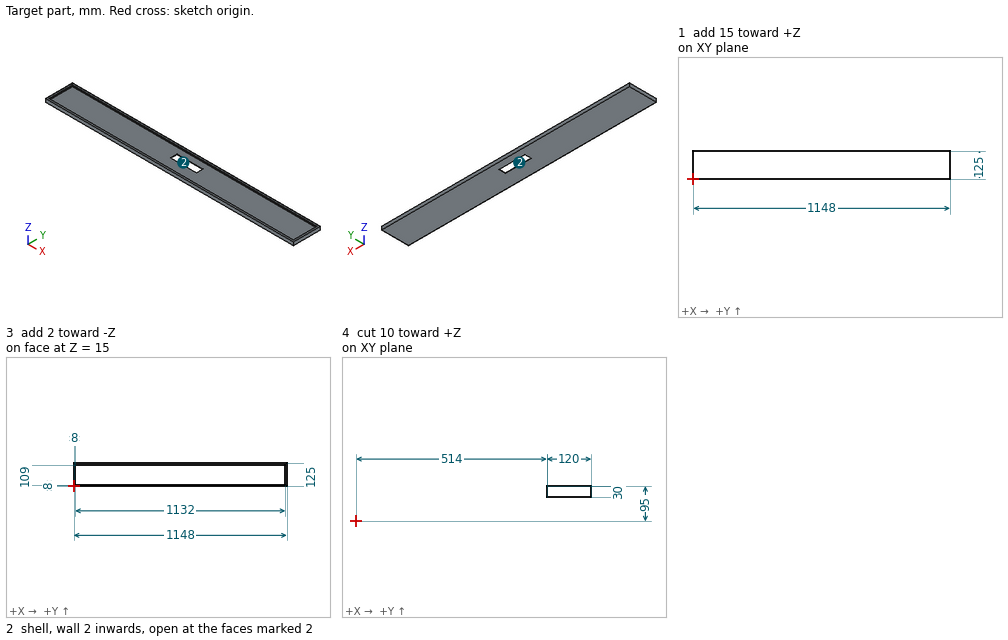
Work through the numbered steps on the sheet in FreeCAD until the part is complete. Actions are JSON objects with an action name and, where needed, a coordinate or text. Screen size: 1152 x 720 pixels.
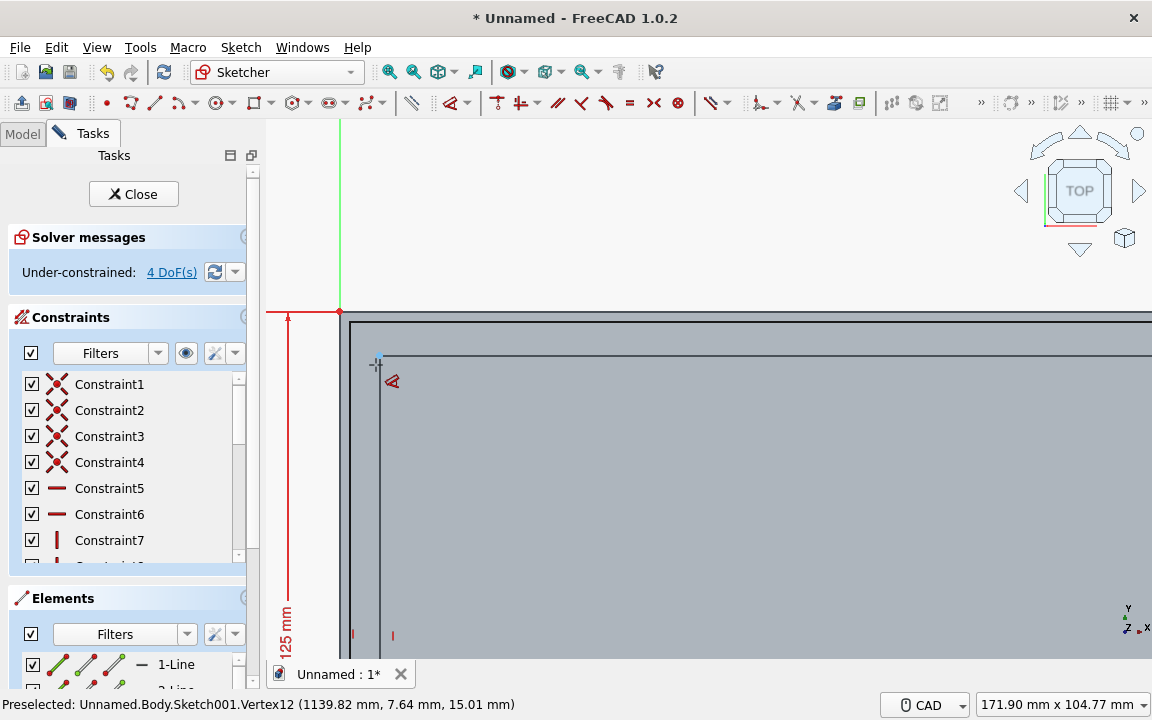
{"action": "left_click", "coordinate": [380, 356]}
{"action": "left_click", "coordinate": [360, 298]}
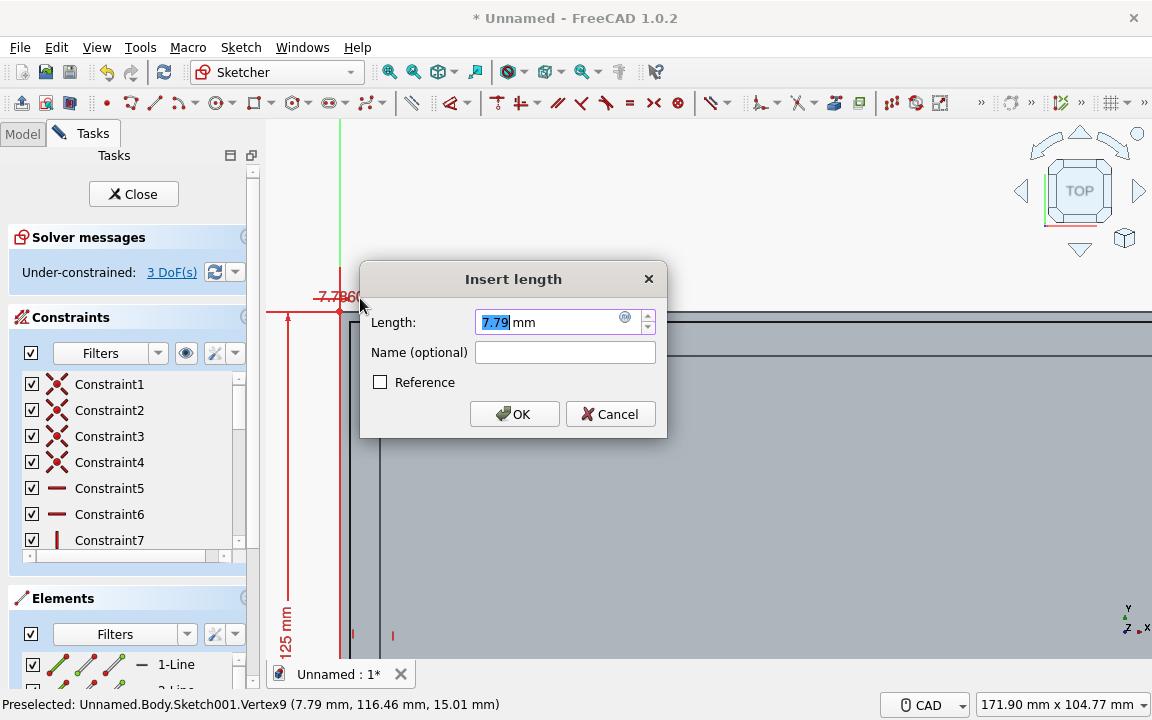
{"action": "type", "text": "8"}
{"action": "key", "text": "Return"}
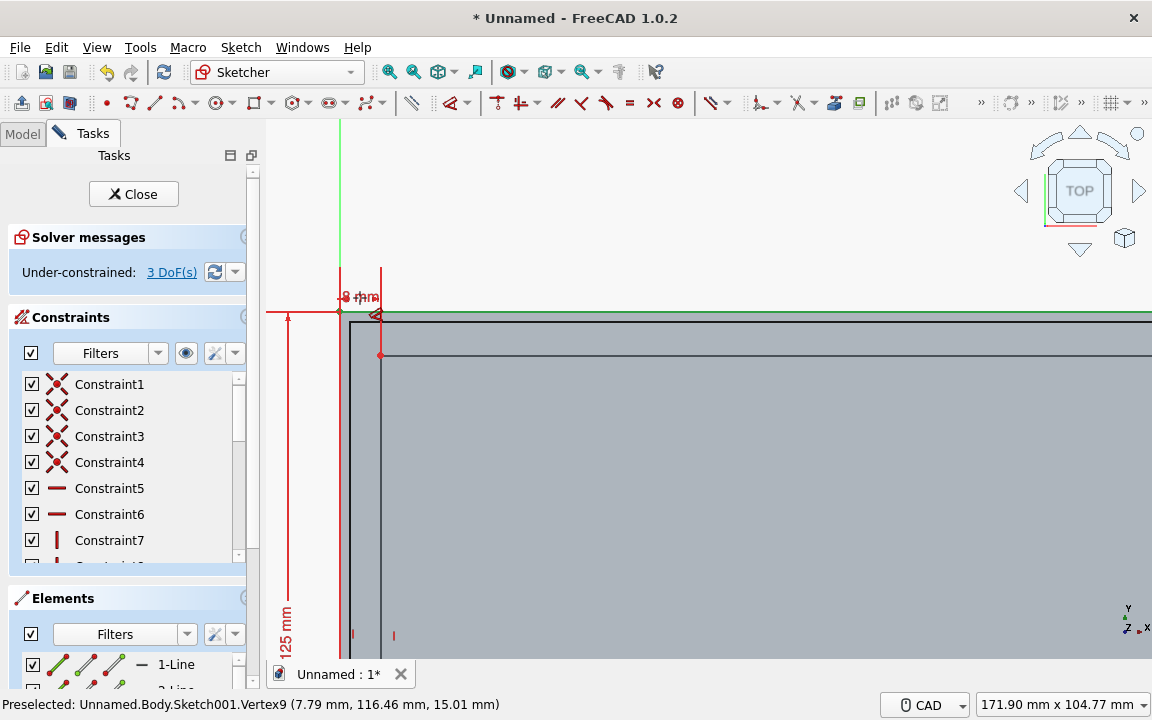
{"action": "scroll", "coordinate": [375, 365], "scroll_direction": "down", "scroll_amount": 12}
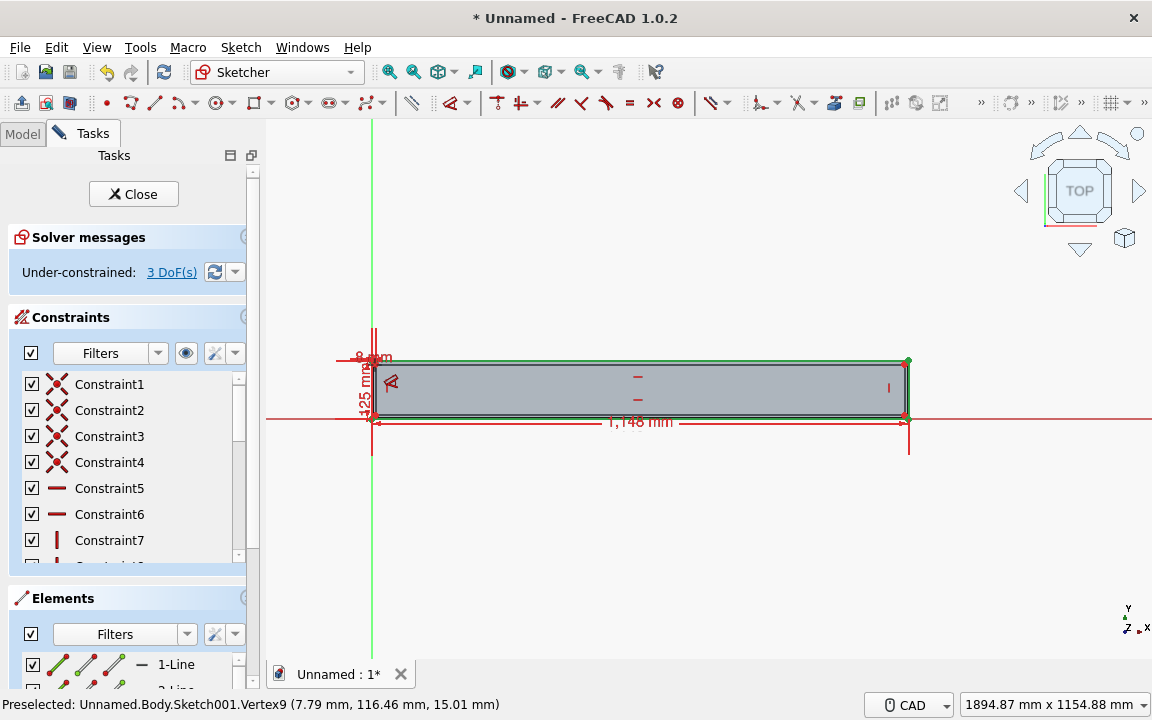
{"action": "scroll", "coordinate": [376, 415], "scroll_direction": "up", "scroll_amount": 12}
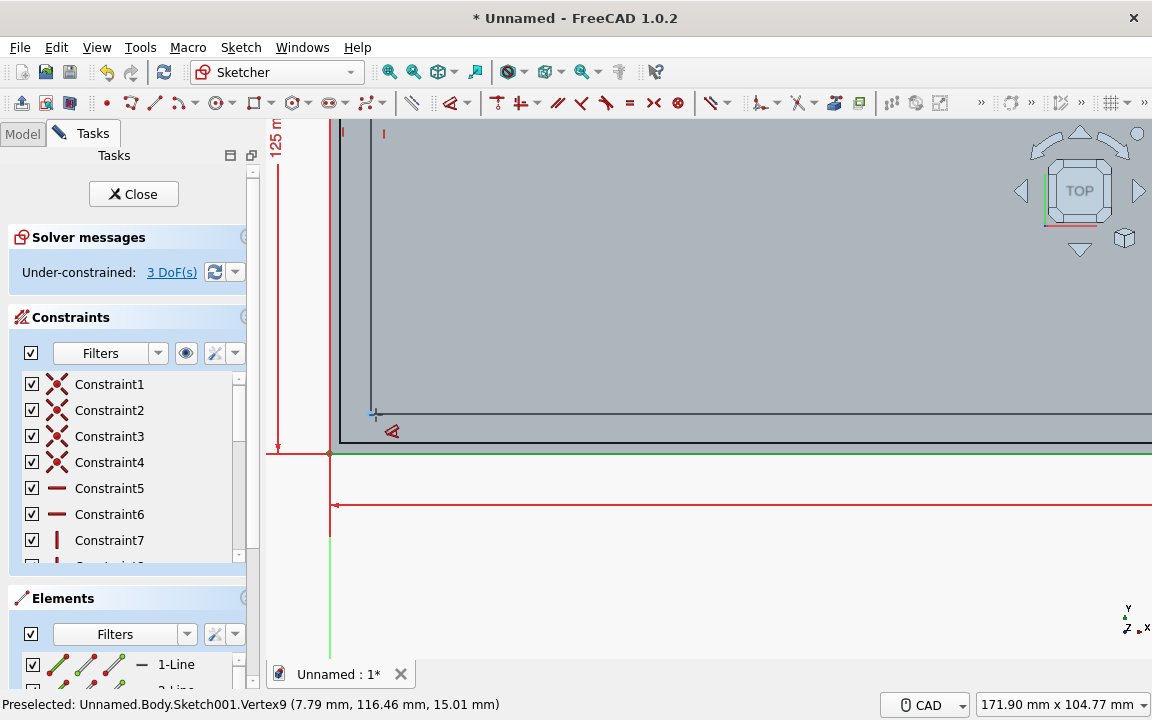
{"action": "left_click", "coordinate": [371, 414]}
{"action": "left_click", "coordinate": [296, 434]}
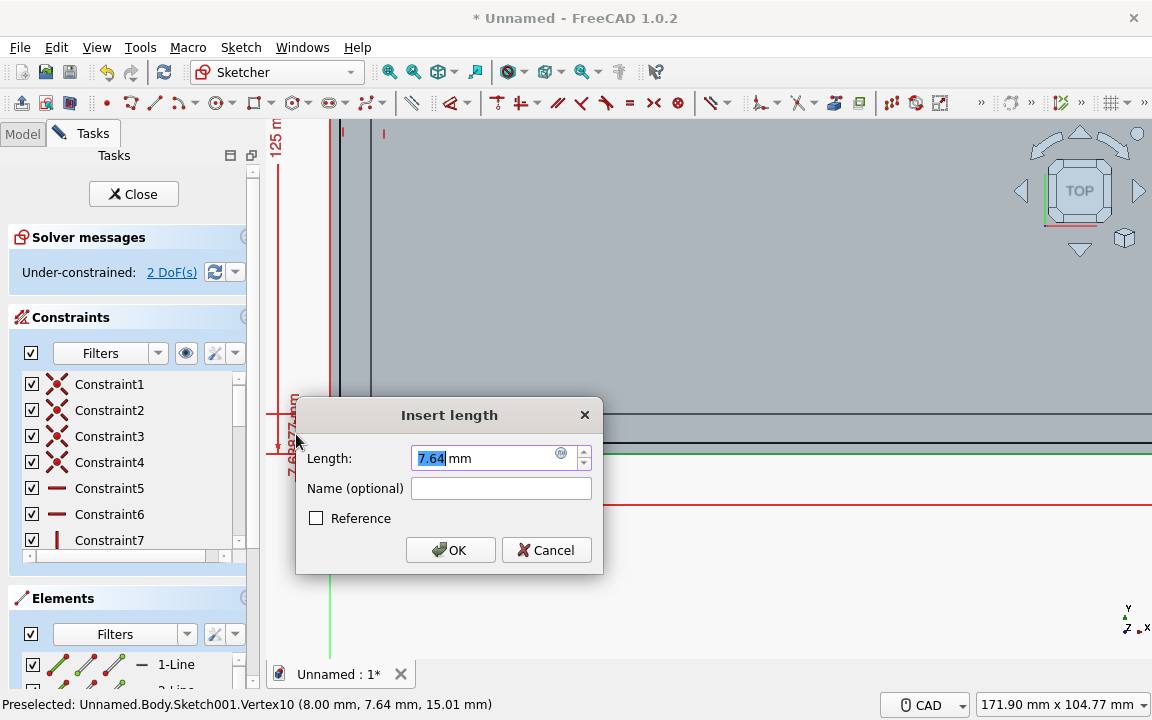
{"action": "type", "text": "8"}
{"action": "key", "text": "Return"}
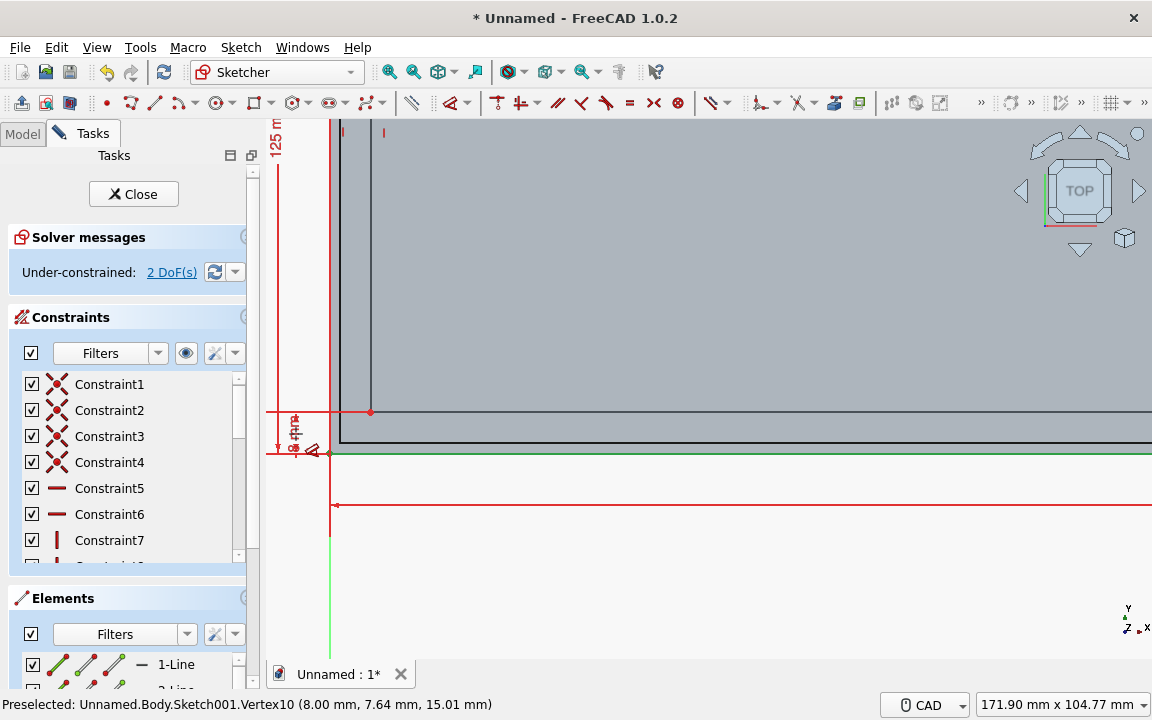
{"action": "scroll", "coordinate": [376, 415], "scroll_direction": "down", "scroll_amount": 12}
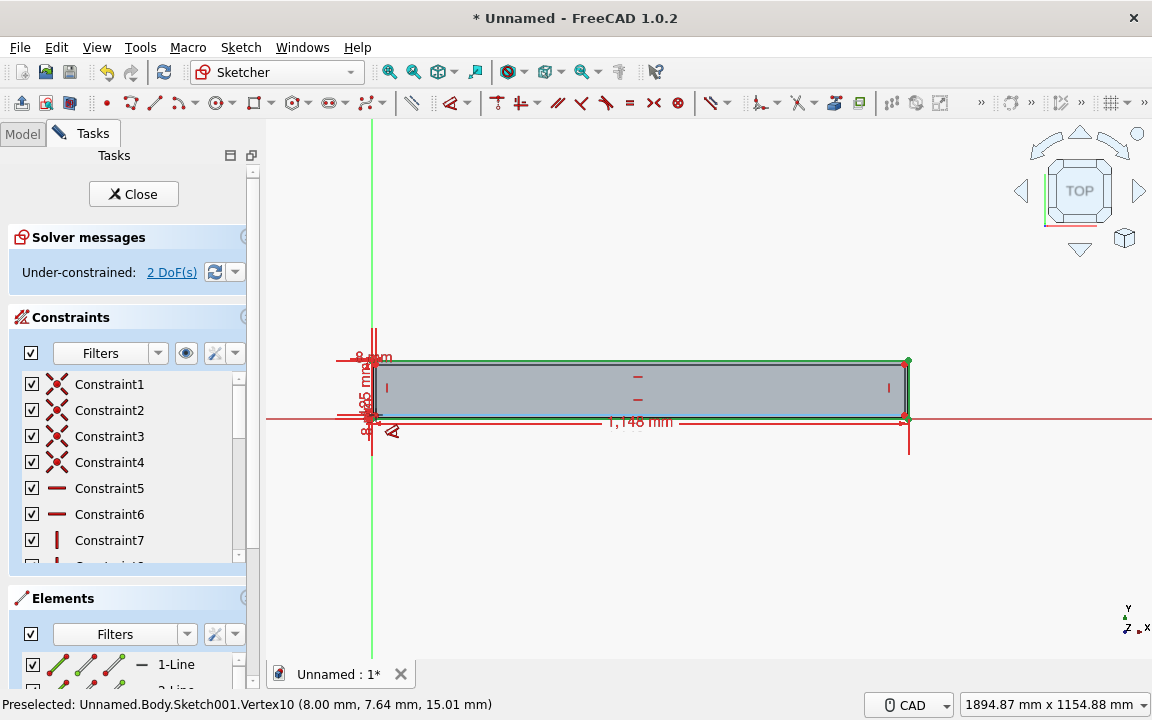
{"action": "scroll", "coordinate": [376, 400], "scroll_direction": "up", "scroll_amount": 7}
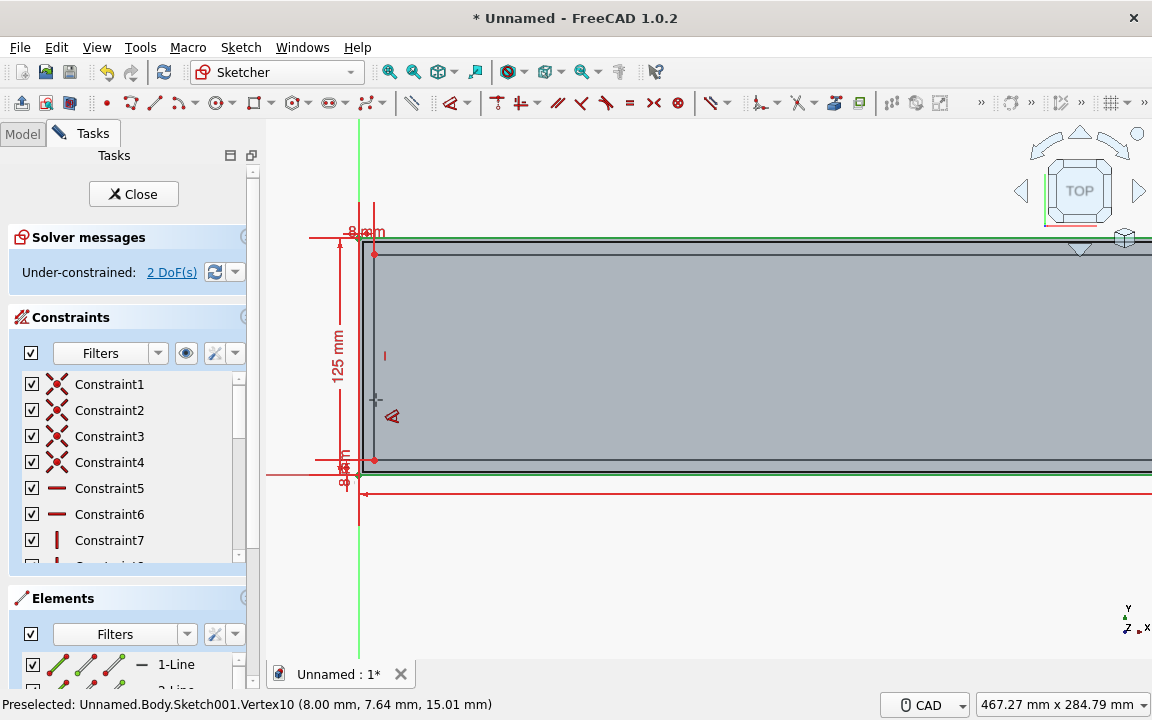
{"action": "left_click", "coordinate": [374, 399]}
{"action": "left_click", "coordinate": [340, 358]}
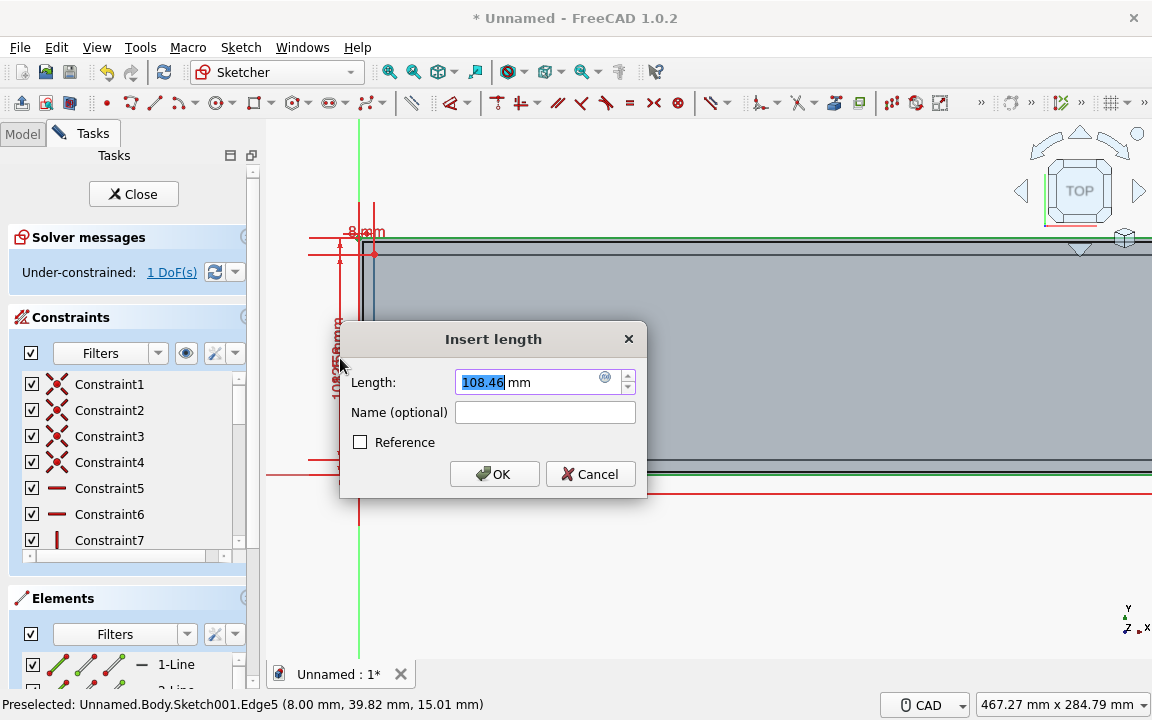
{"action": "type", "text": "109"}
{"action": "key", "text": "Return"}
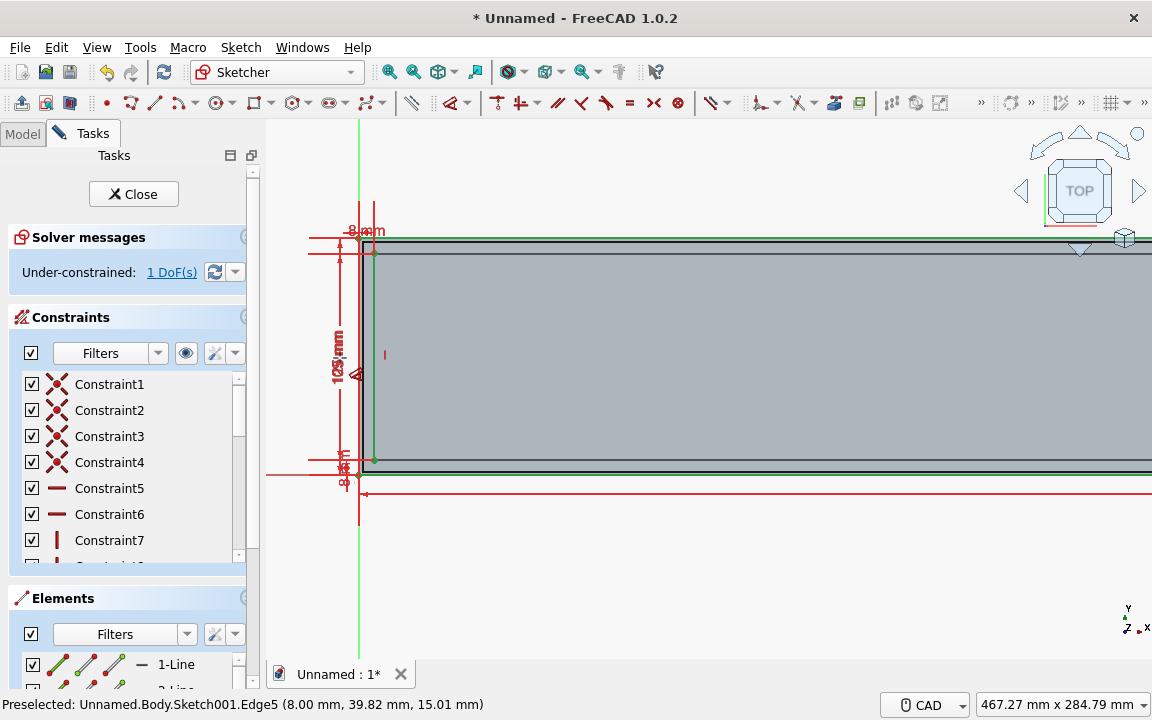
{"action": "left_click", "coordinate": [803, 460]}
{"action": "left_click", "coordinate": [681, 494]}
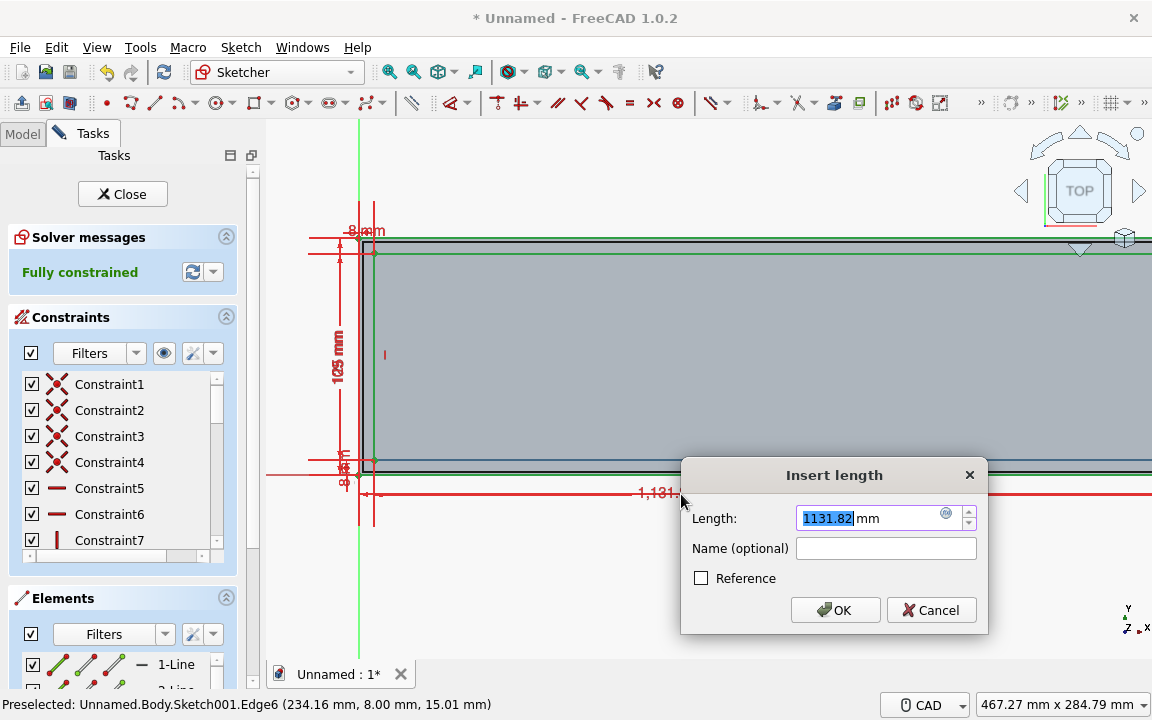
{"action": "type", "text": "1132"}
{"action": "key", "text": "Return"}
{"action": "key", "text": "Escape"}